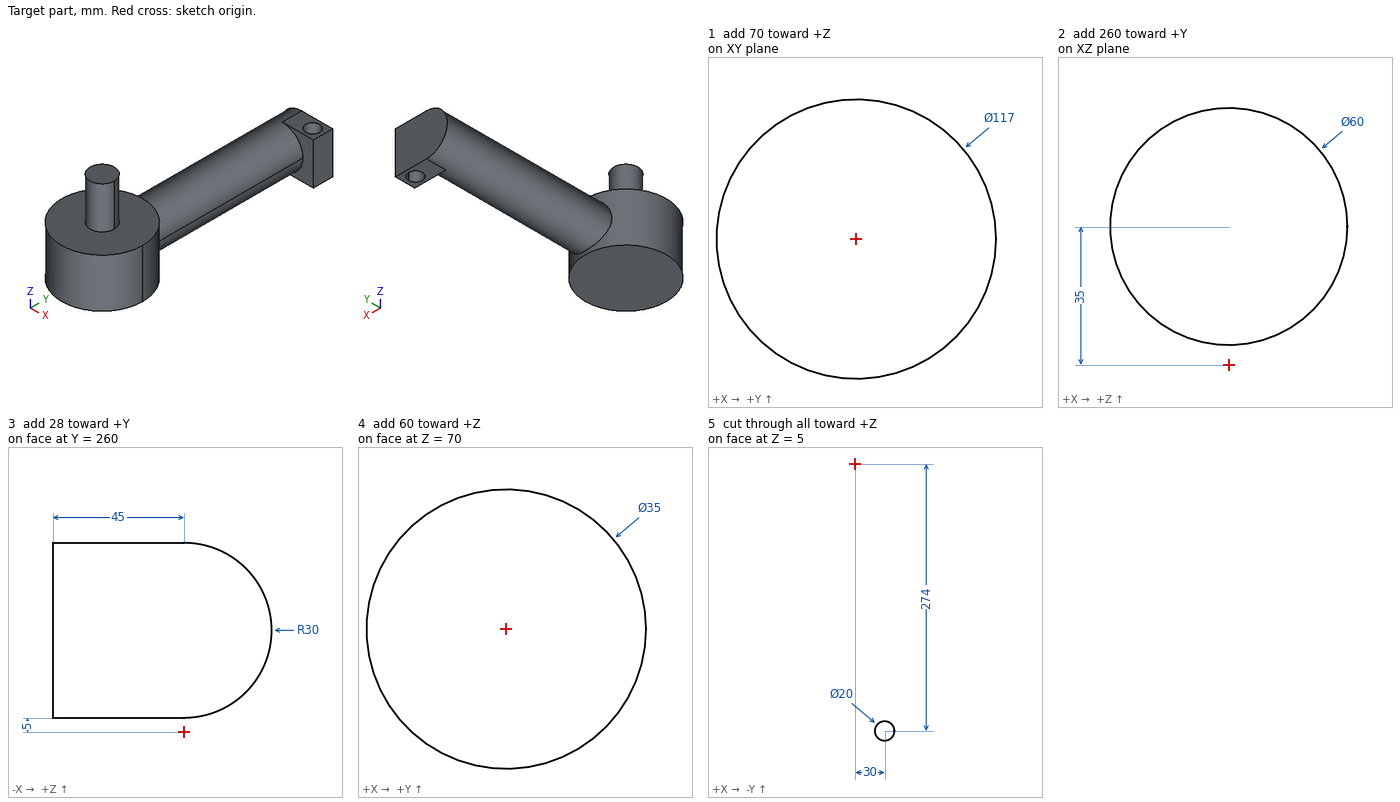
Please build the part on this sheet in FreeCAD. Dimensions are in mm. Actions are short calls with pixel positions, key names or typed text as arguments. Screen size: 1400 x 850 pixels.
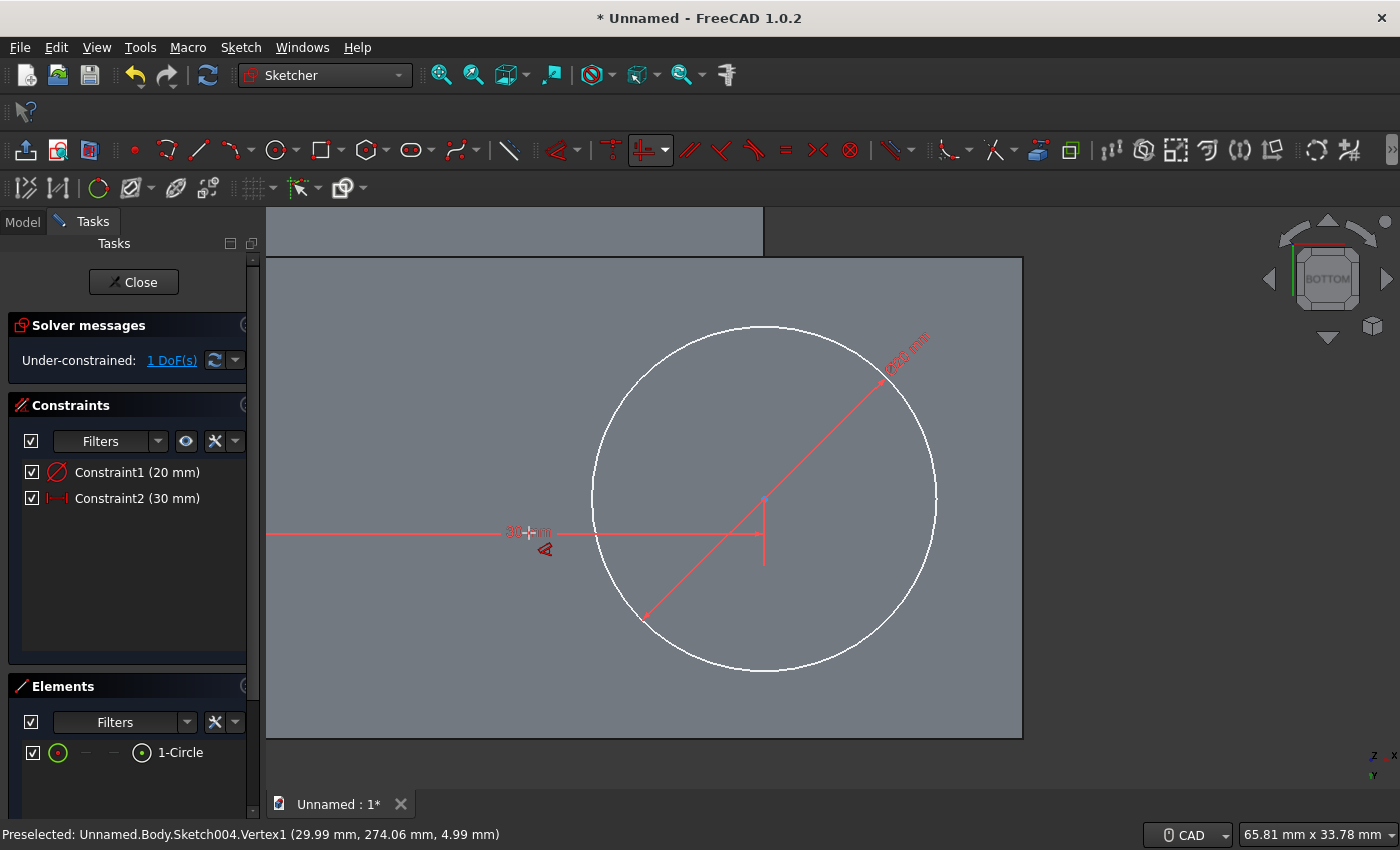
click(764, 499)
click(798, 367)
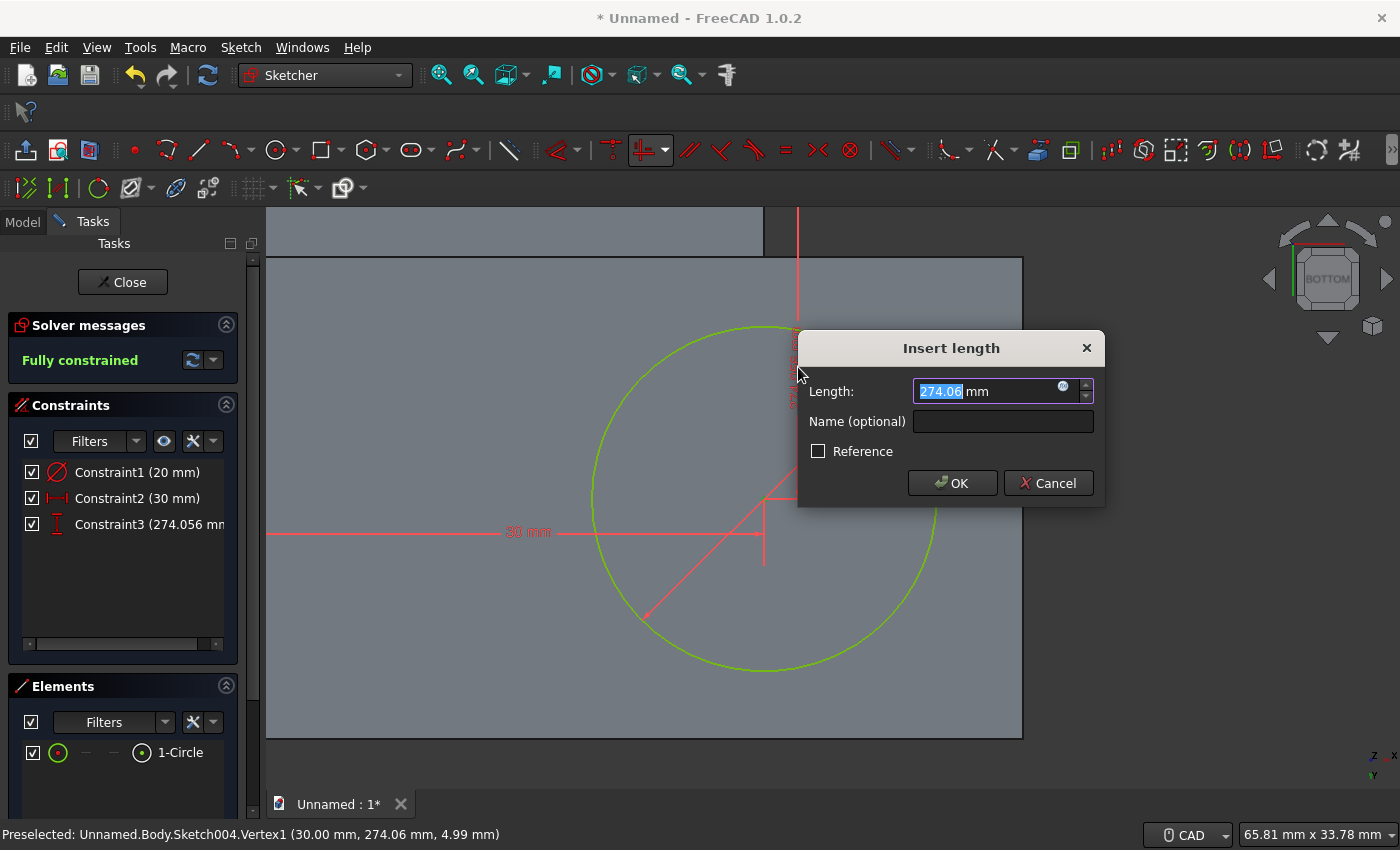
text(274)
key(Return)
key(Escape)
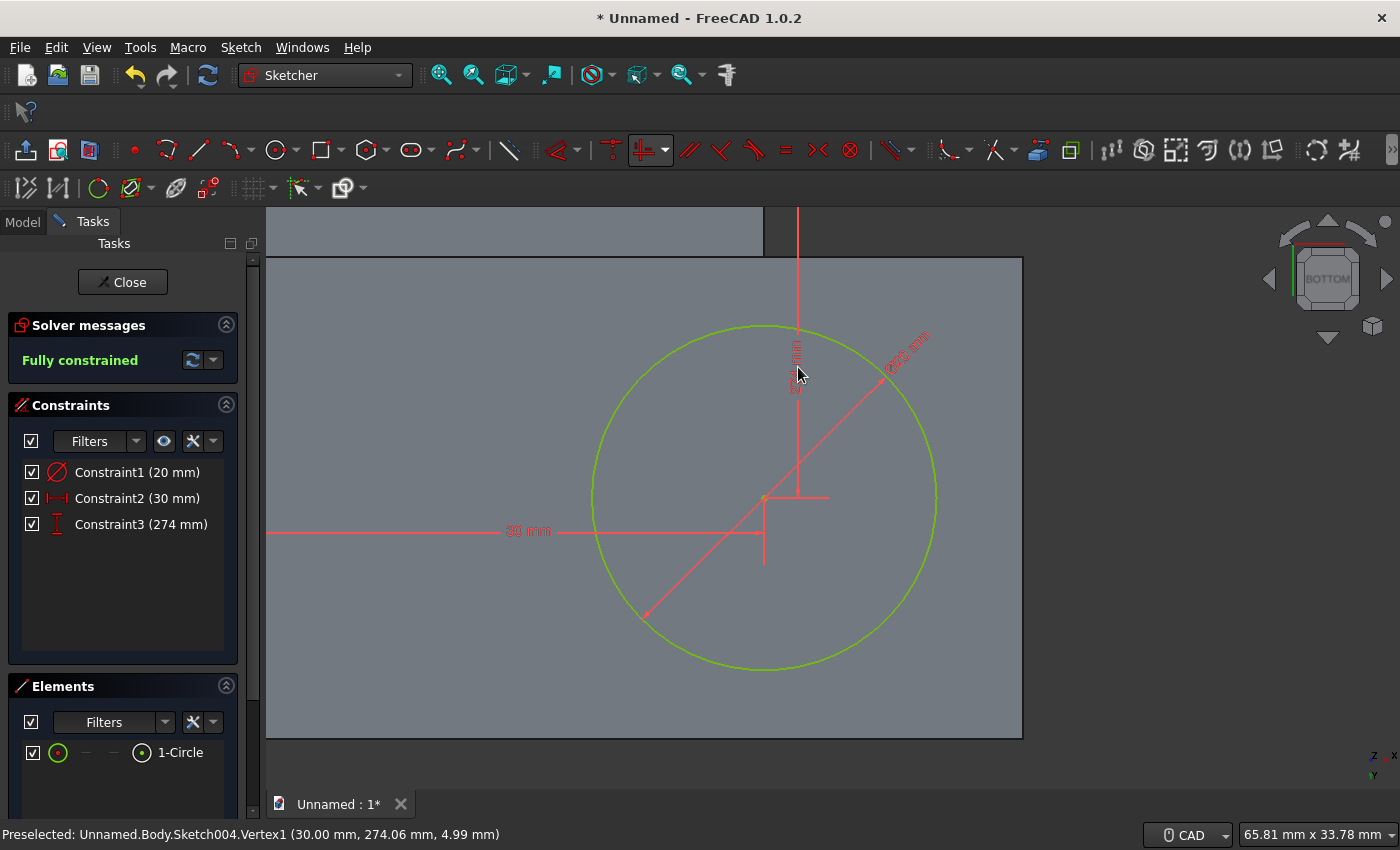
click(123, 282)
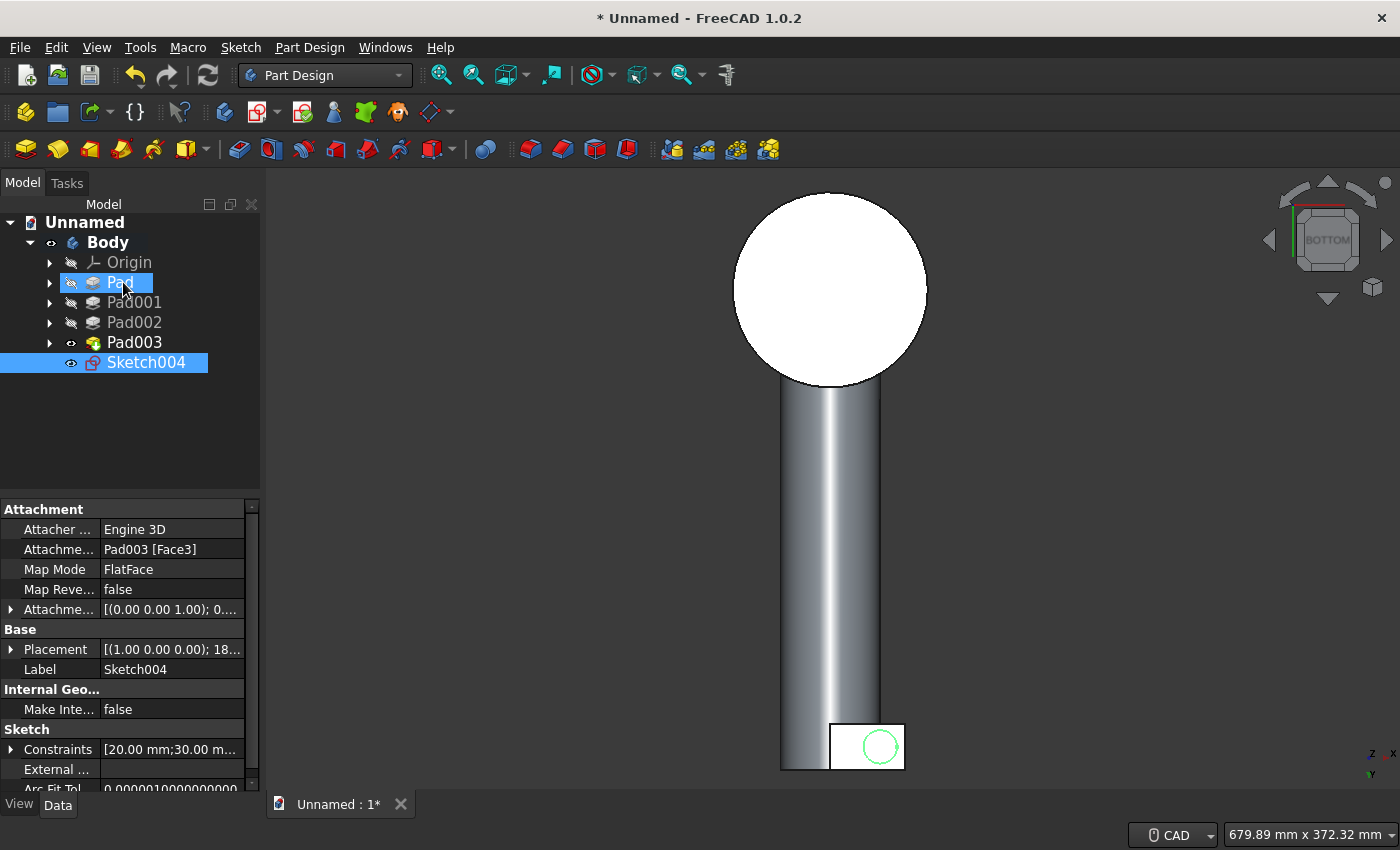
click(240, 150)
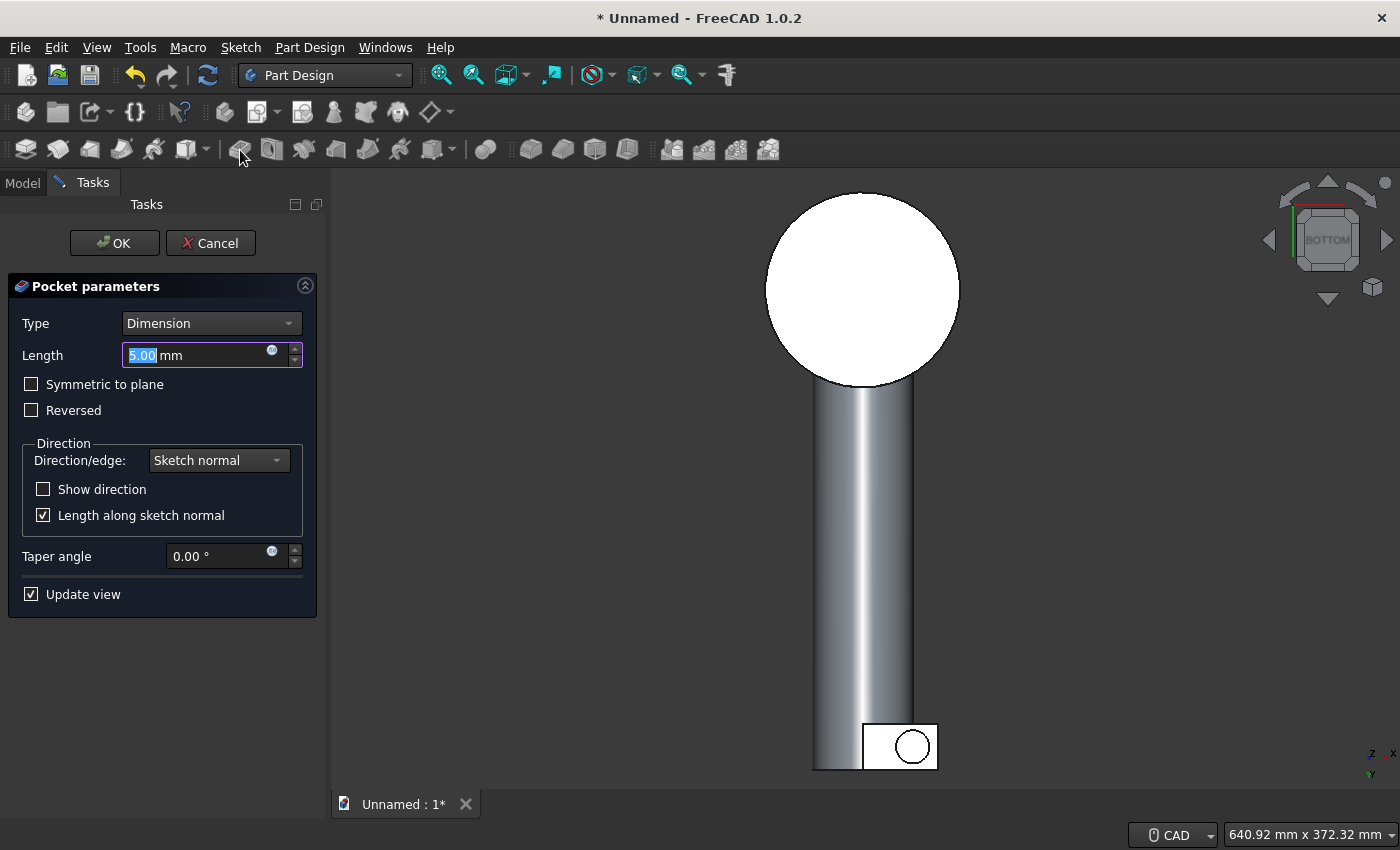
click(212, 324)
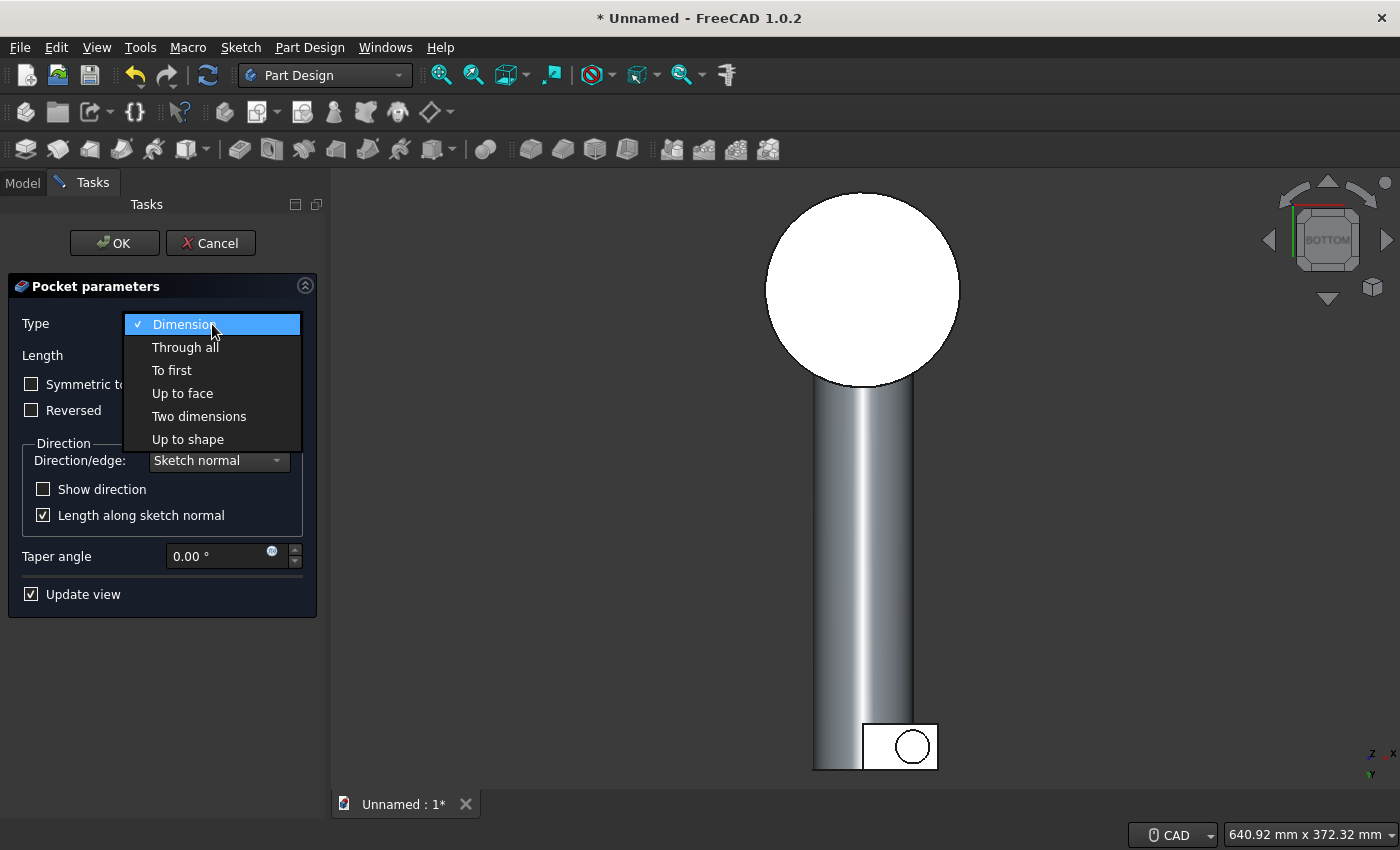
click(212, 348)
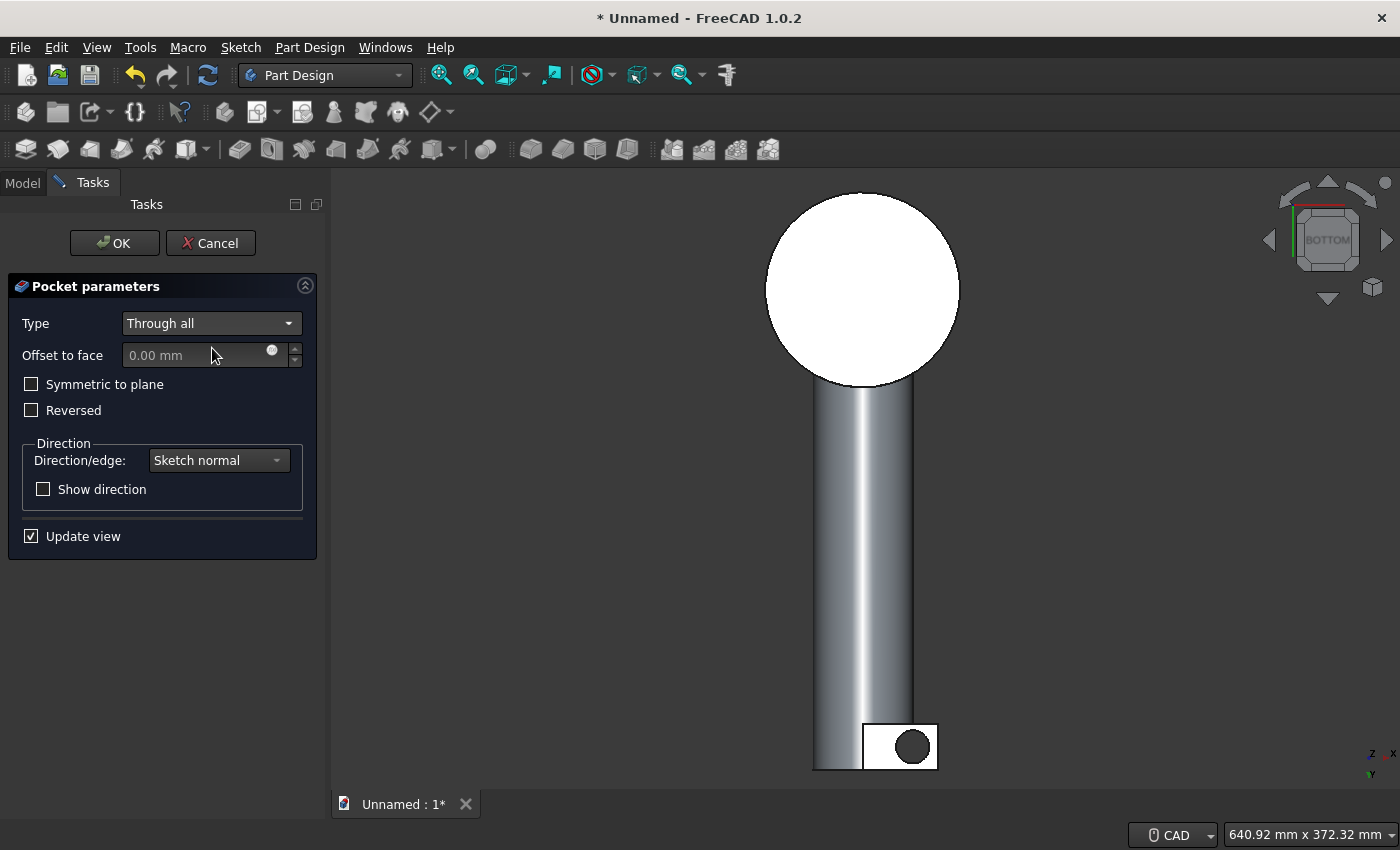
click(115, 243)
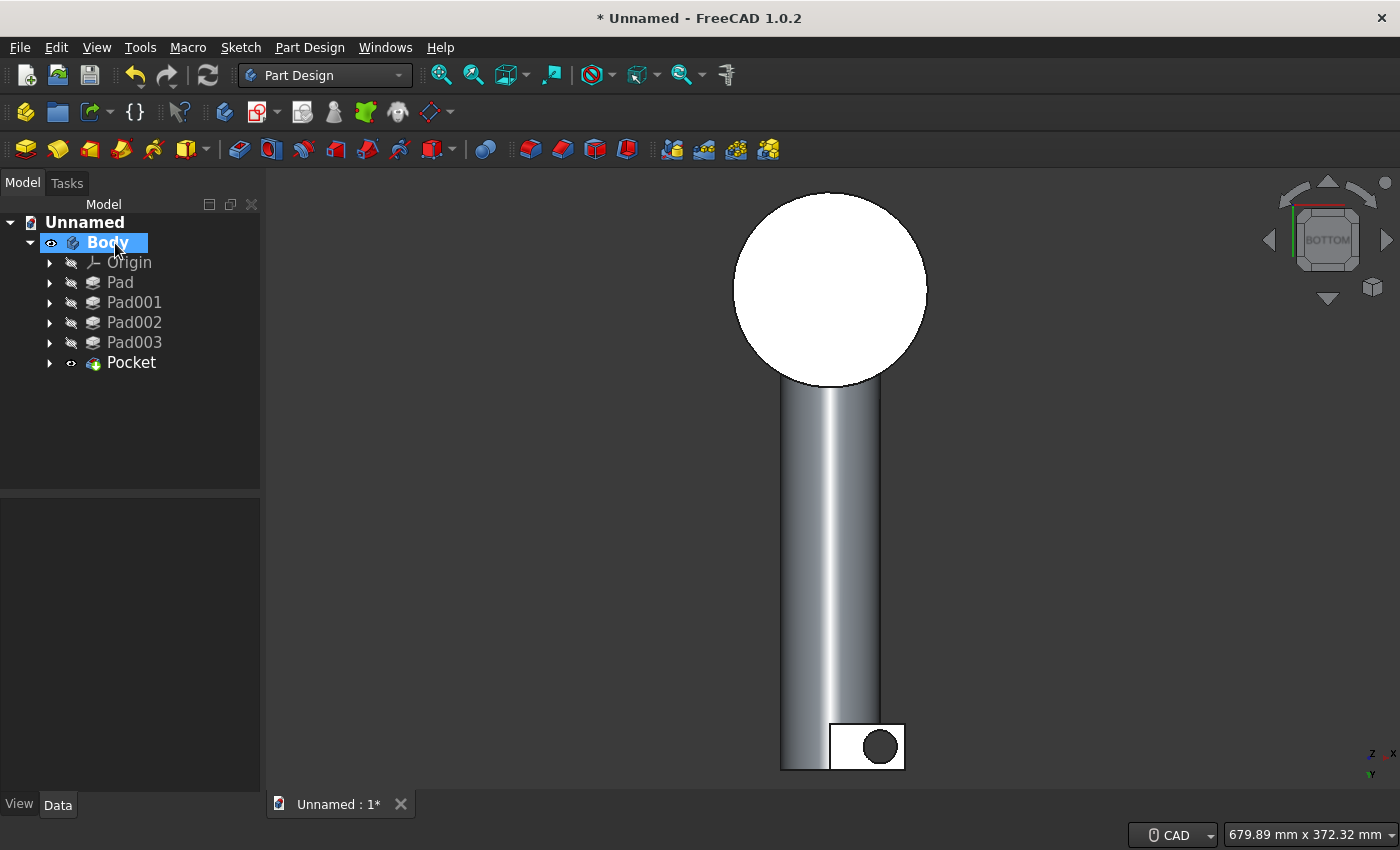
key(0)